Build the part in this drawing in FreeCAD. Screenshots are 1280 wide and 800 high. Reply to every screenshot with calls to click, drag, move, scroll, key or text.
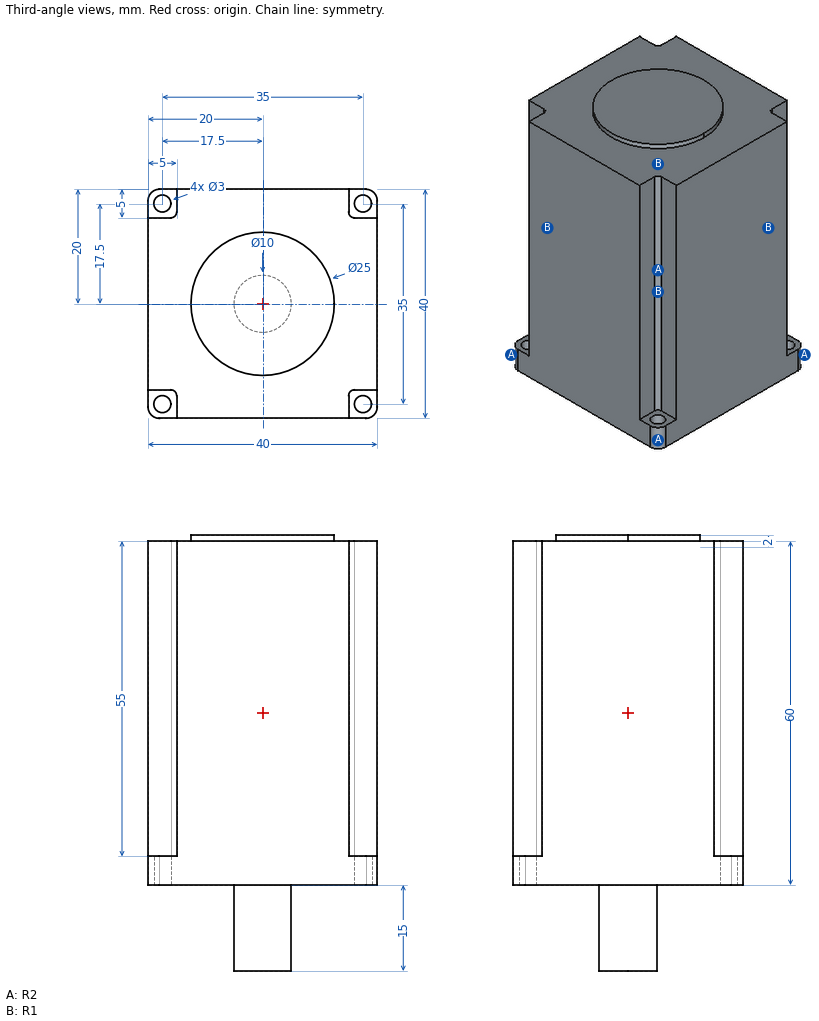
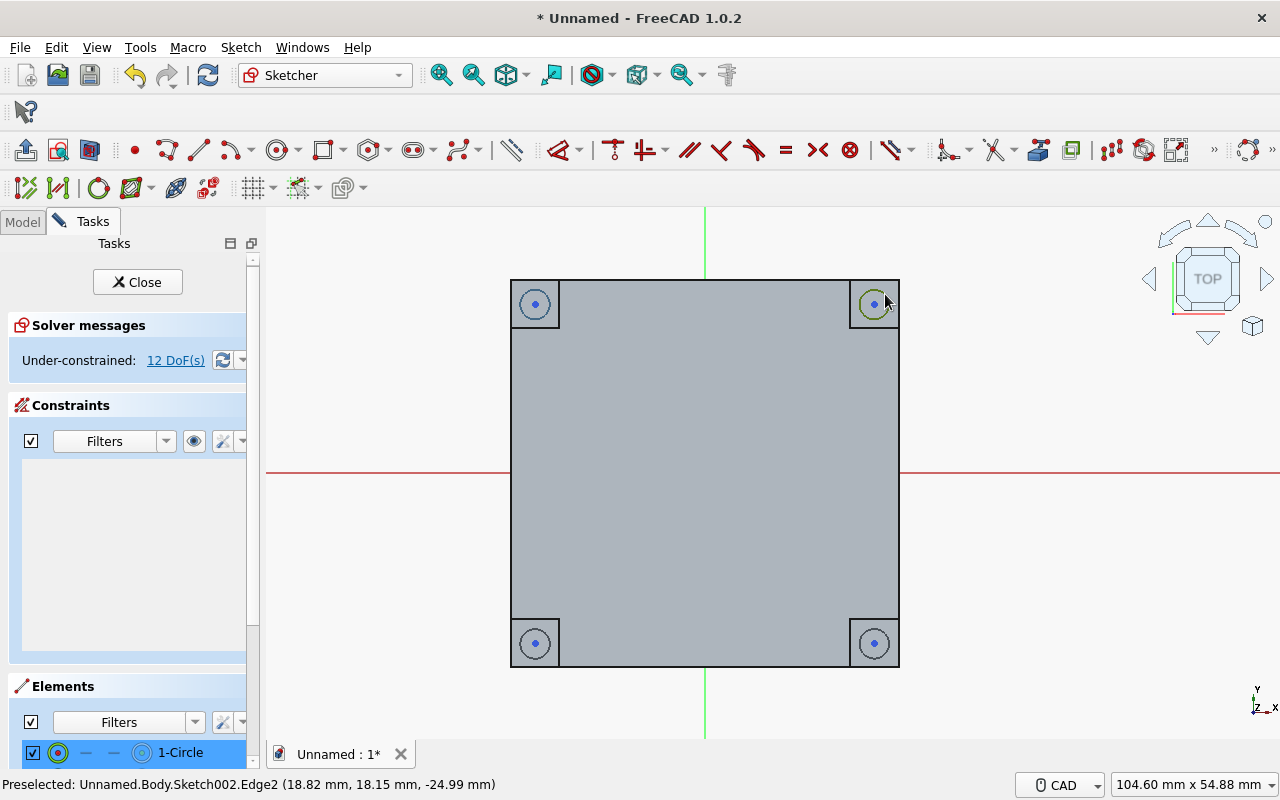
click(885, 633)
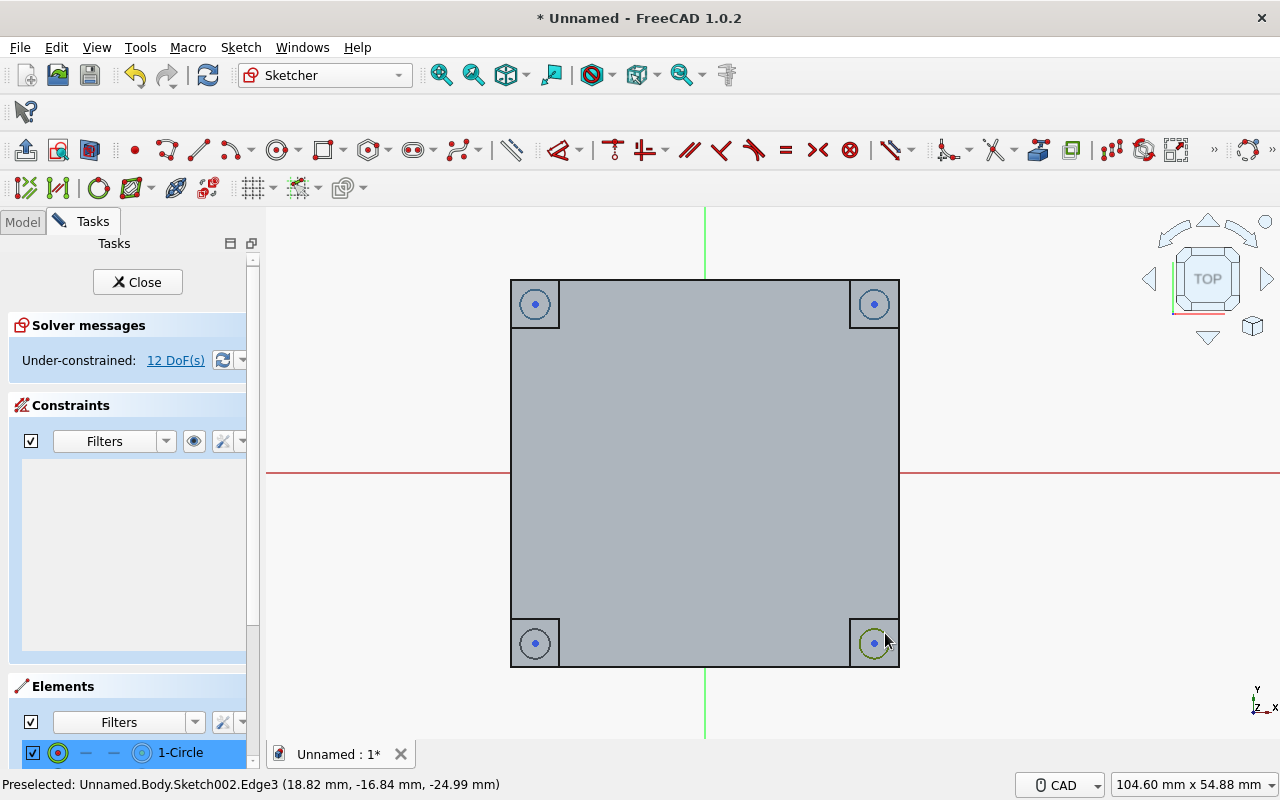
click(546, 633)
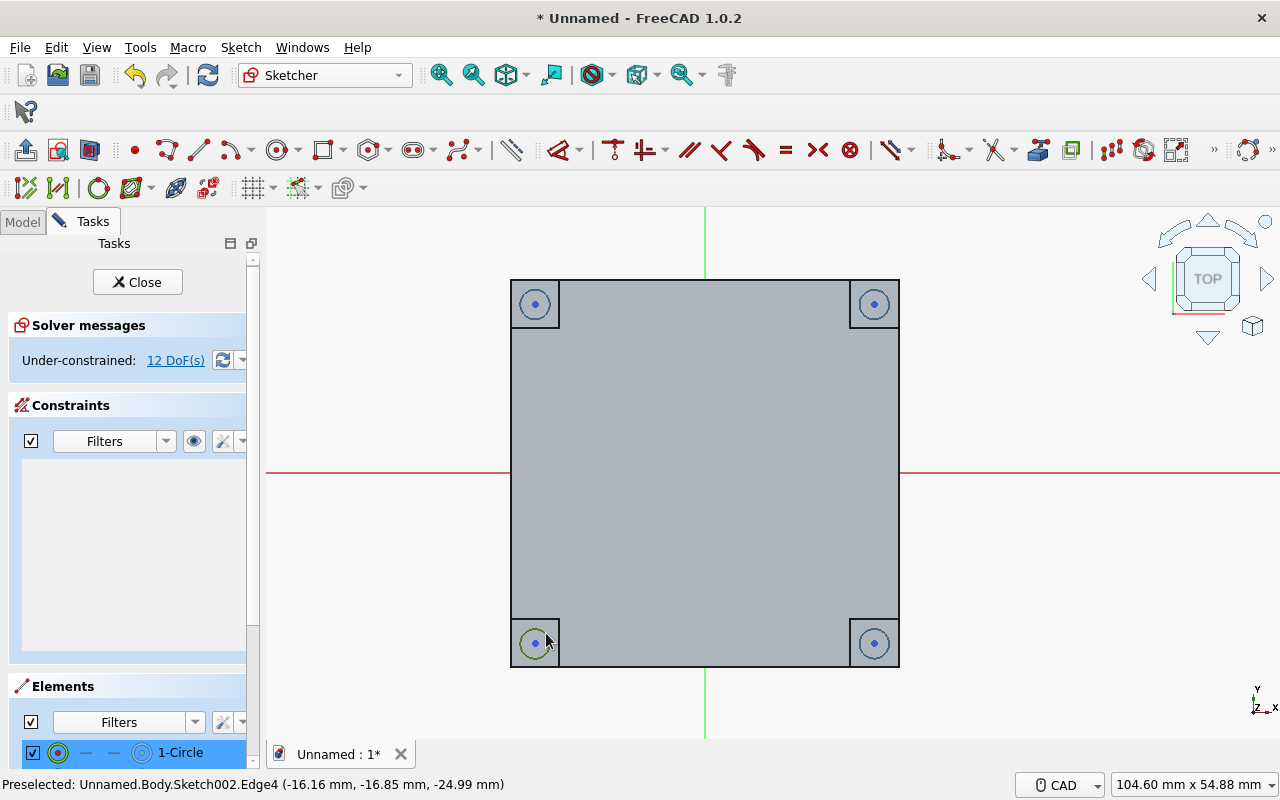
click(786, 150)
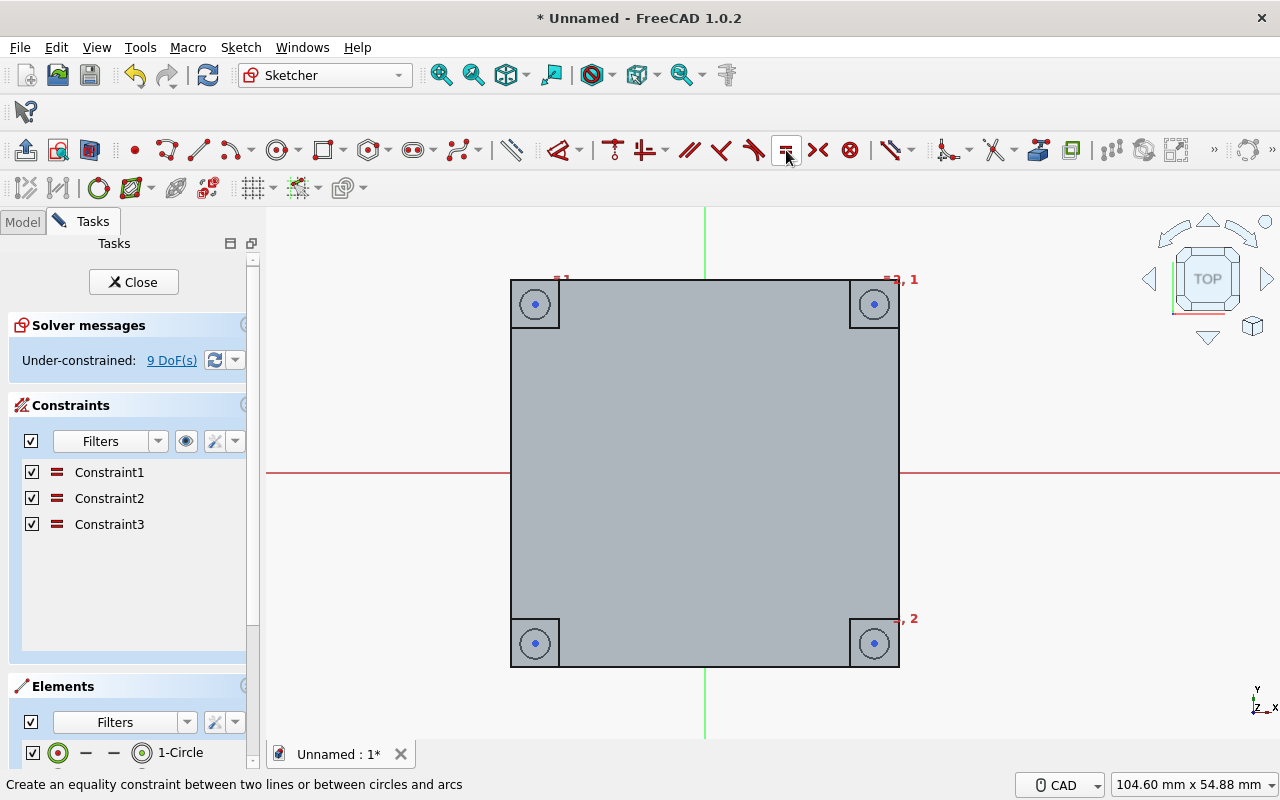
click(535, 305)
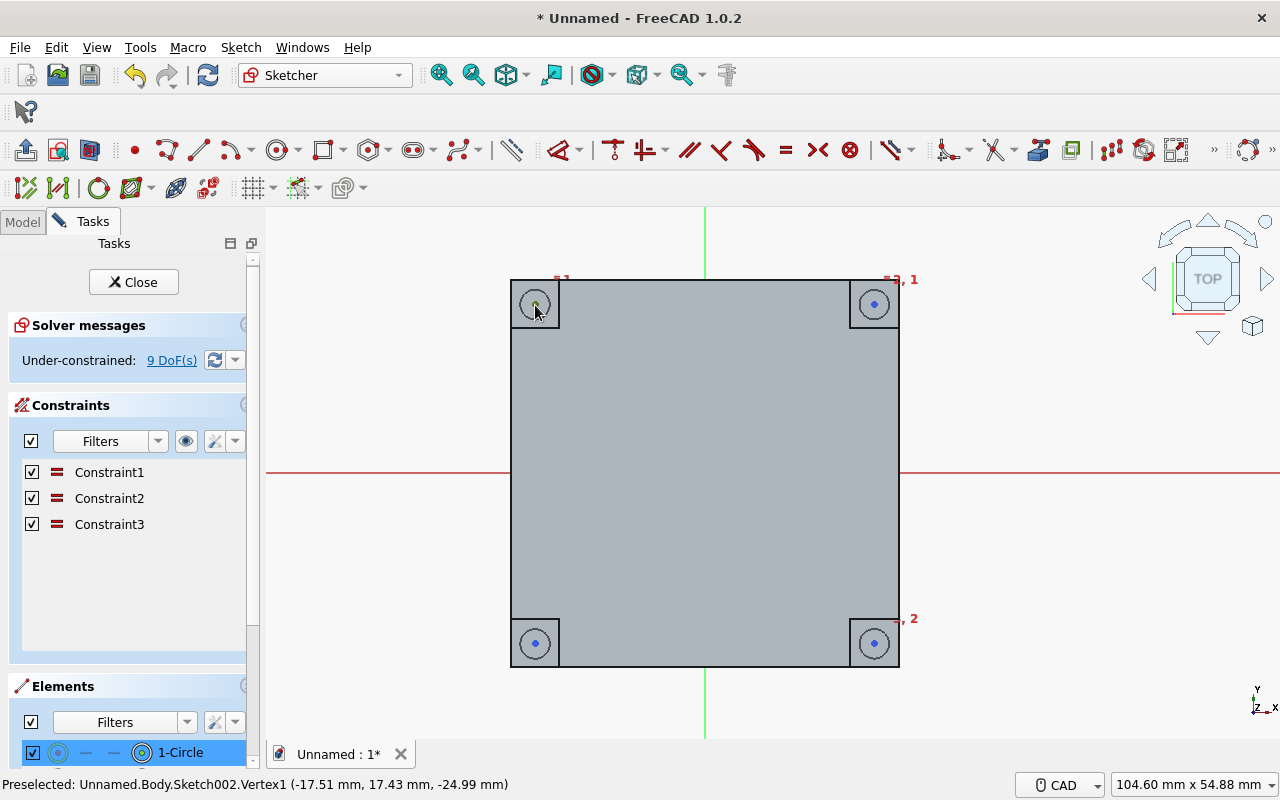
click(874, 305)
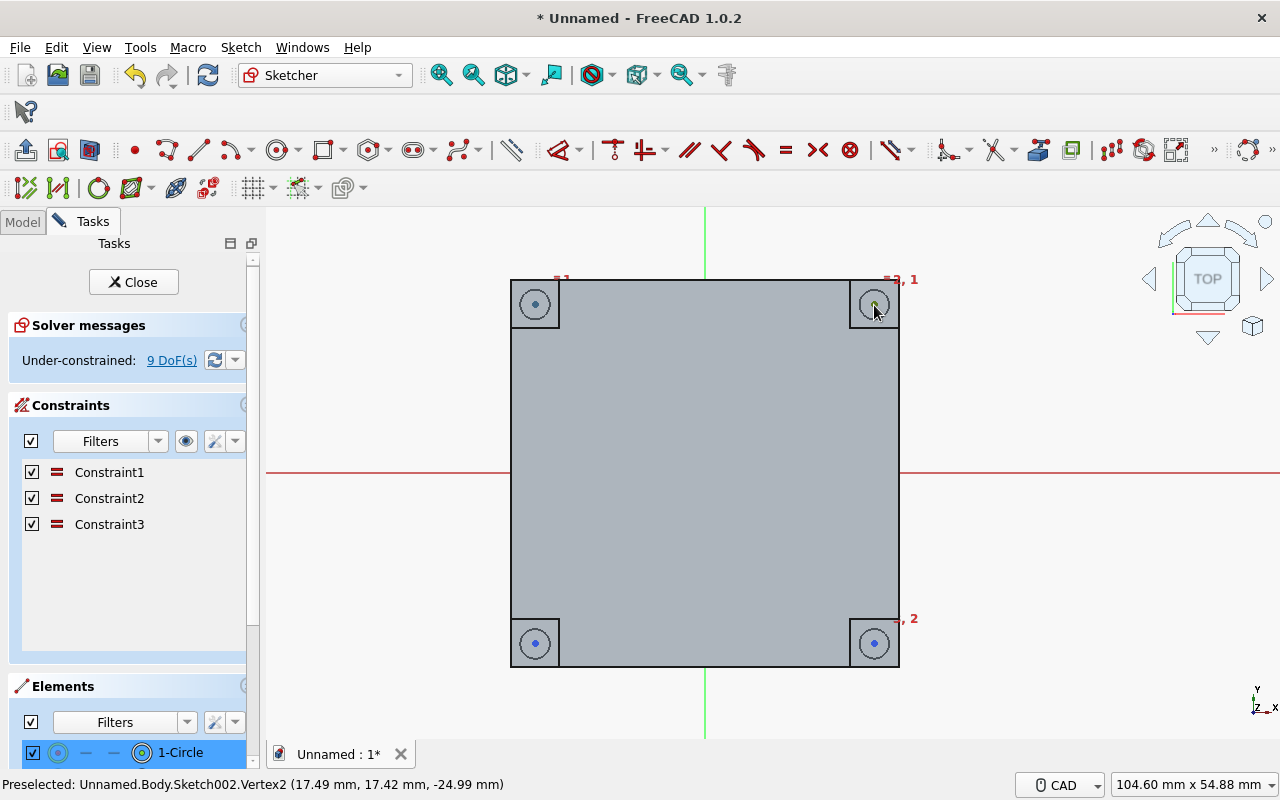
click(668, 150)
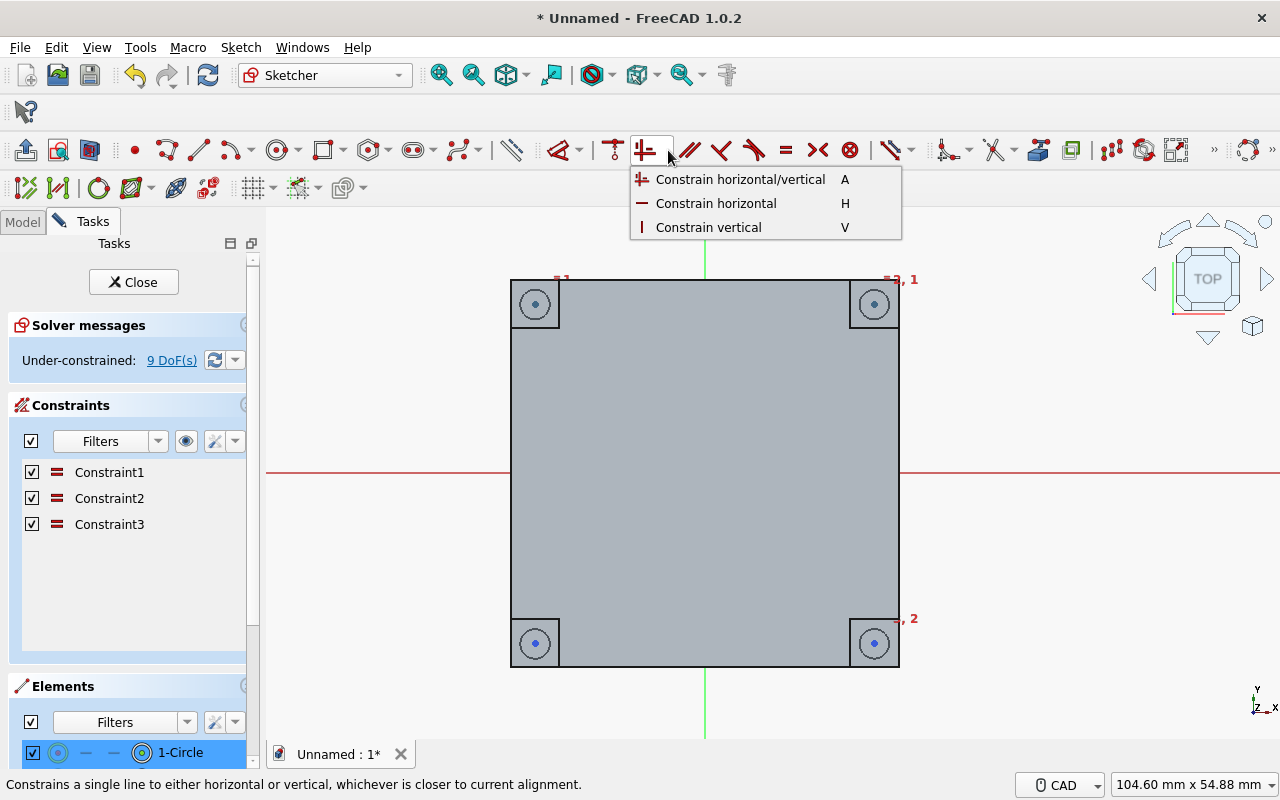
click(766, 203)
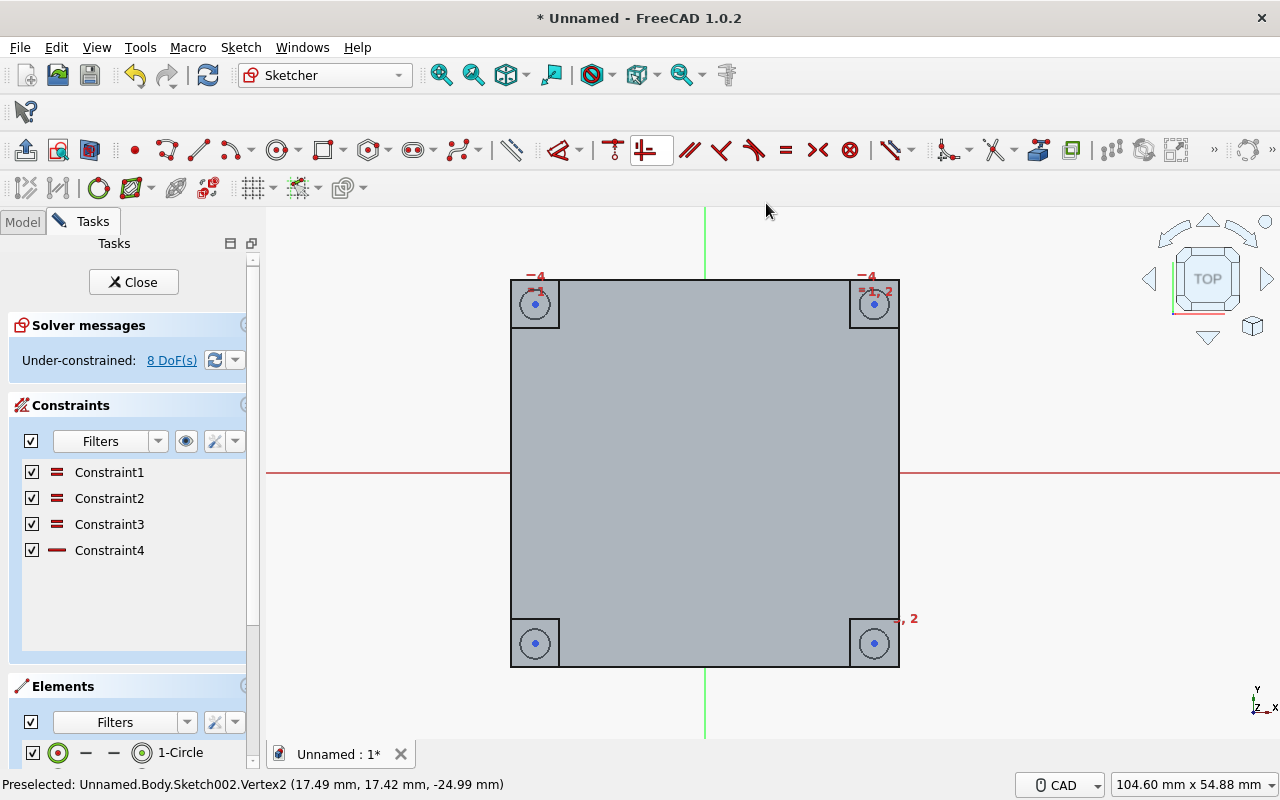
click(874, 305)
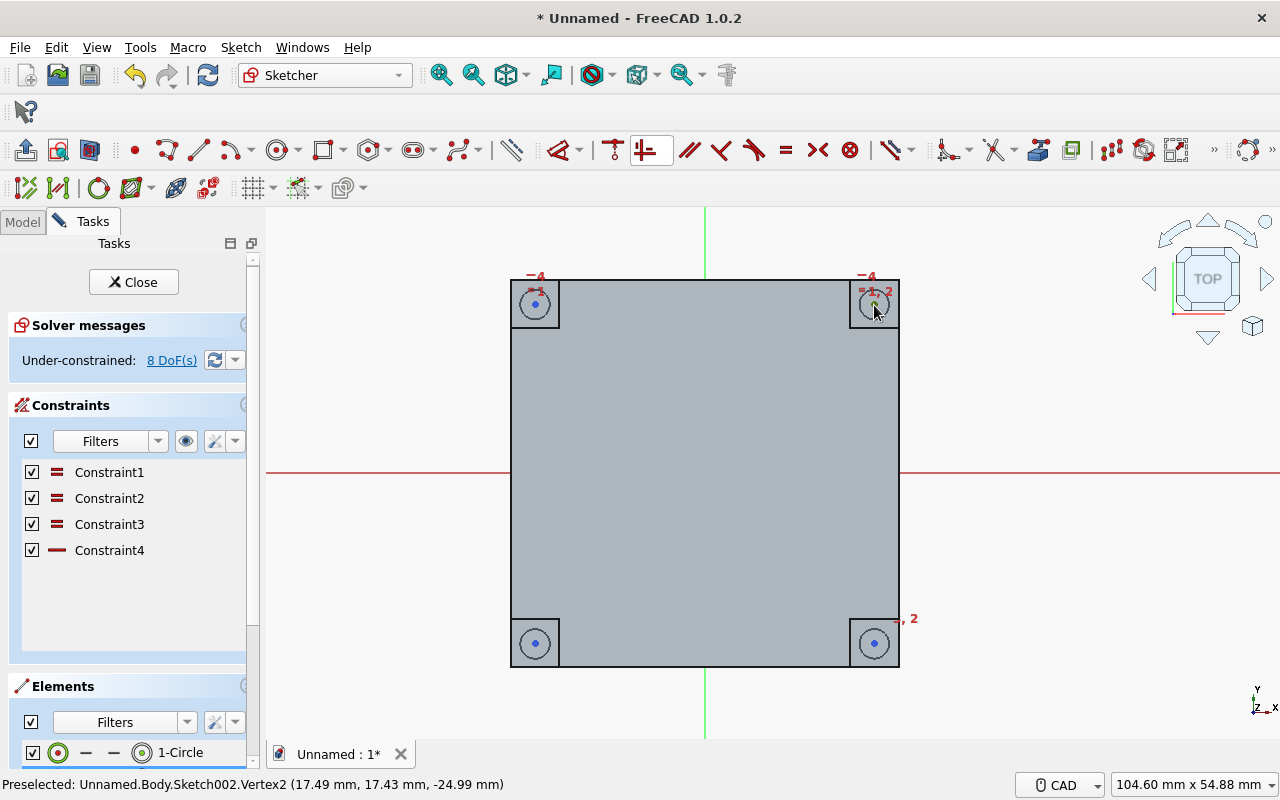
click(874, 644)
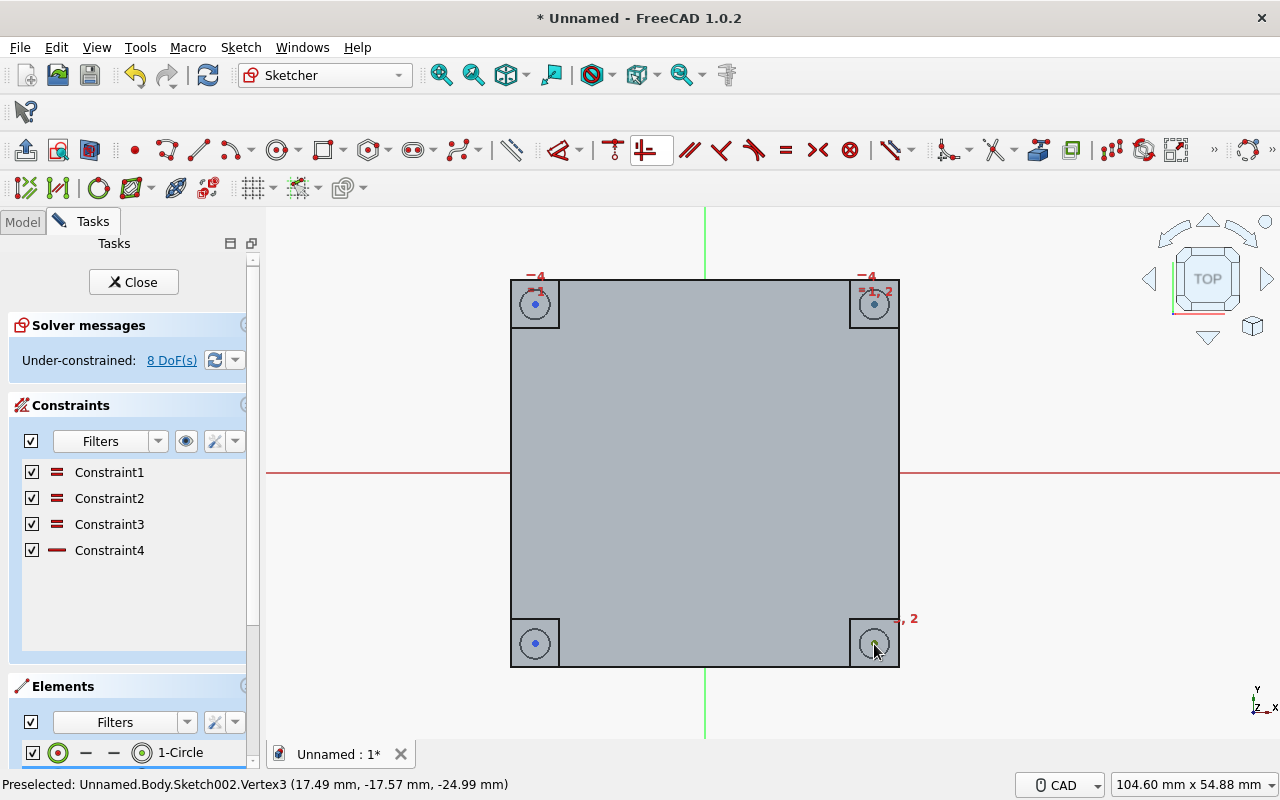
click(668, 150)